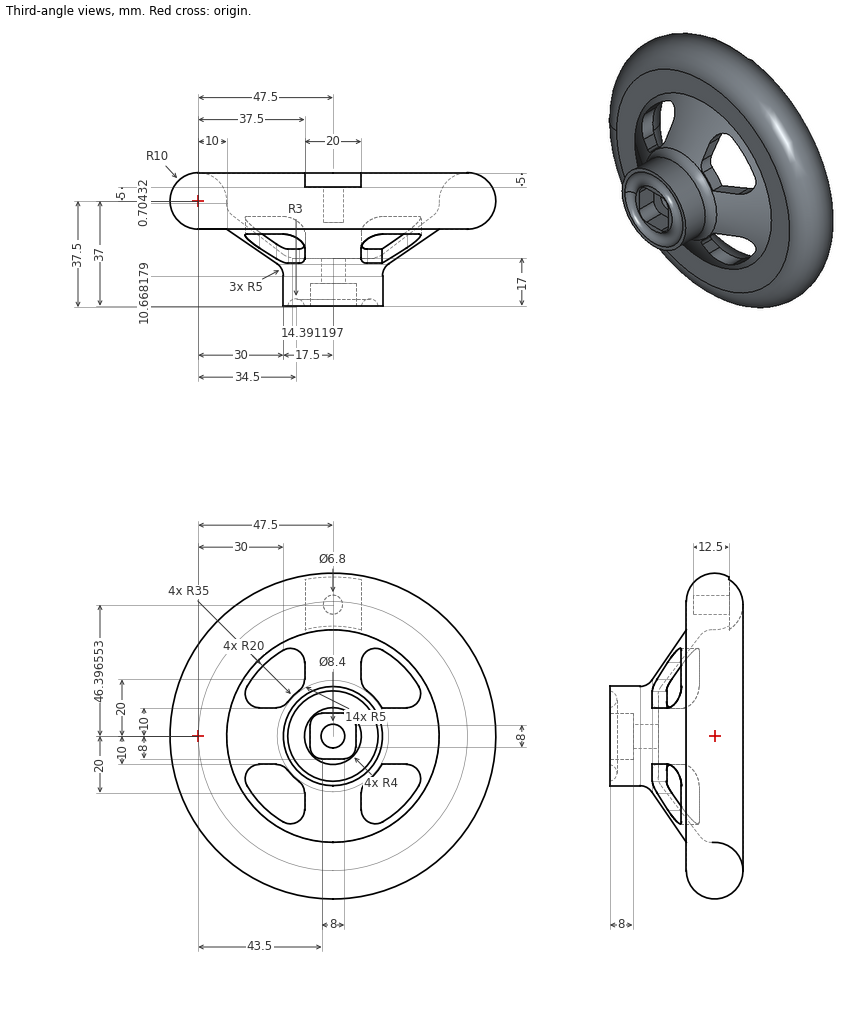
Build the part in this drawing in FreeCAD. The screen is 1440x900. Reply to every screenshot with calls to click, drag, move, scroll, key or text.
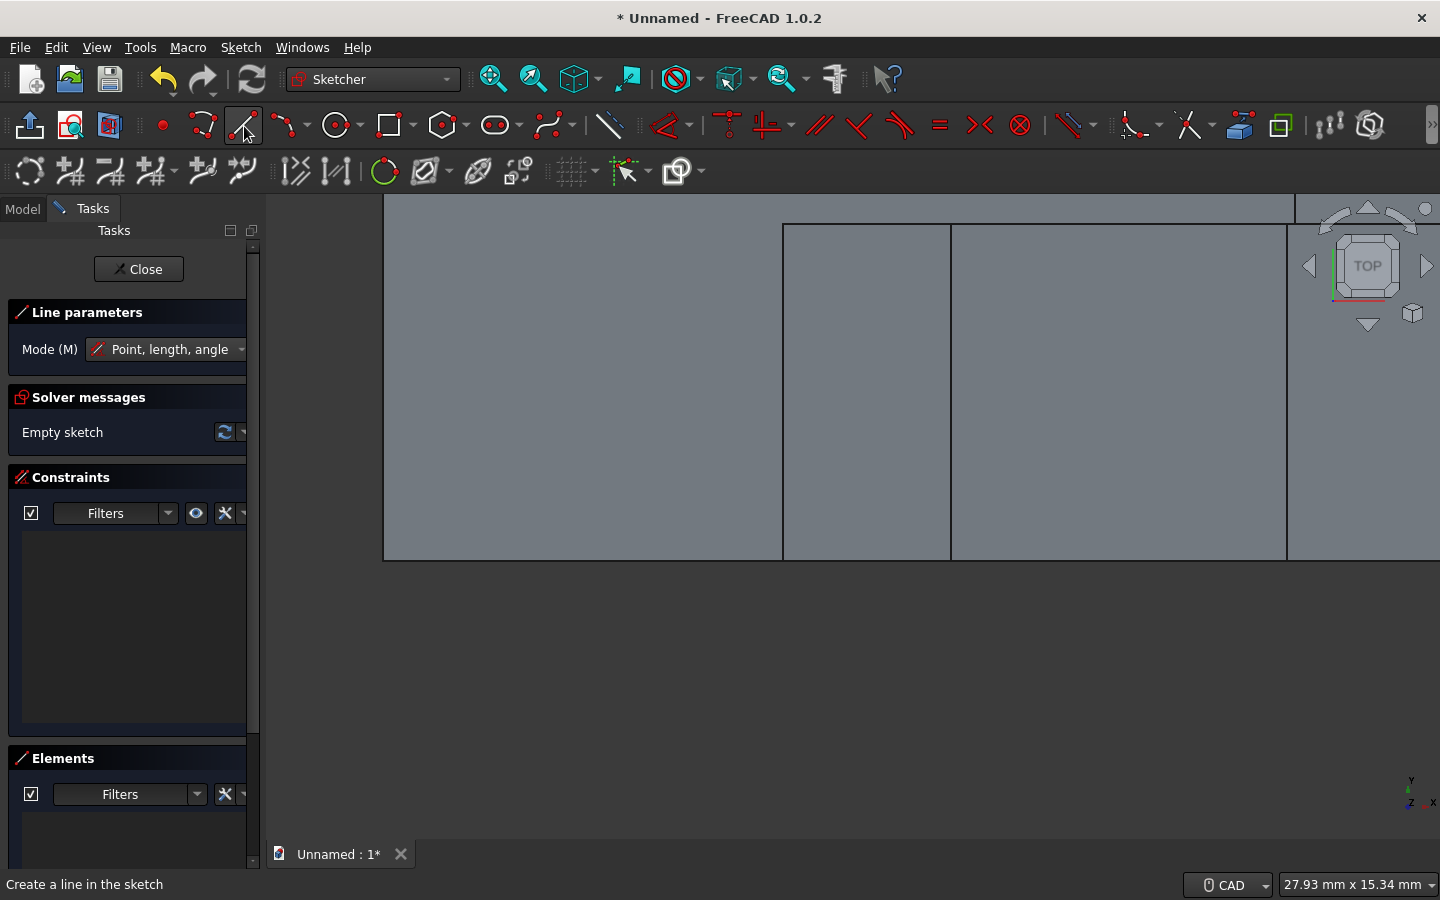
click(448, 561)
click(697, 561)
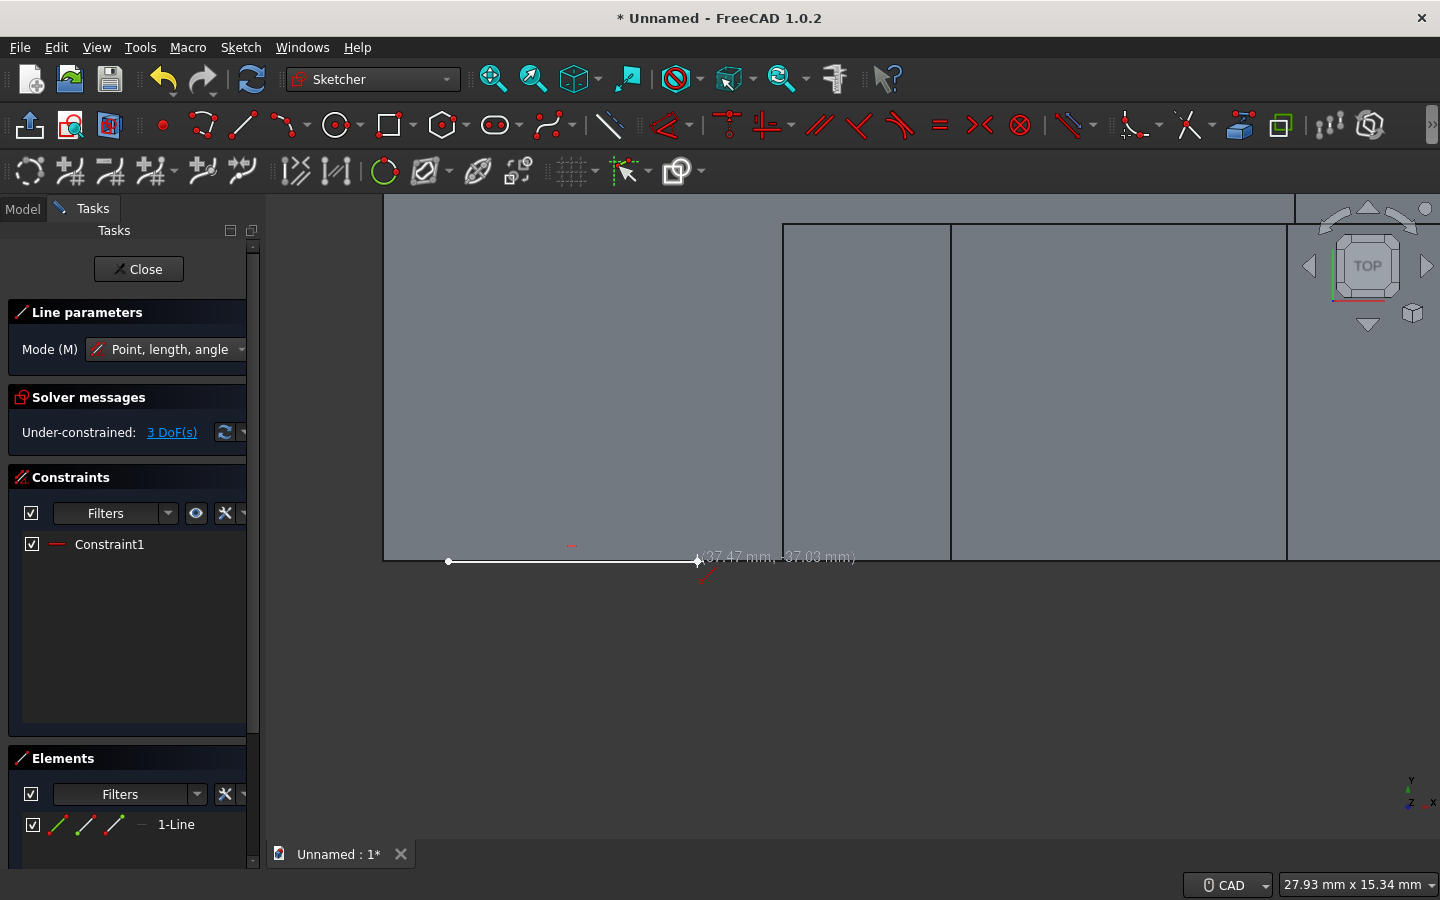
click(284, 126)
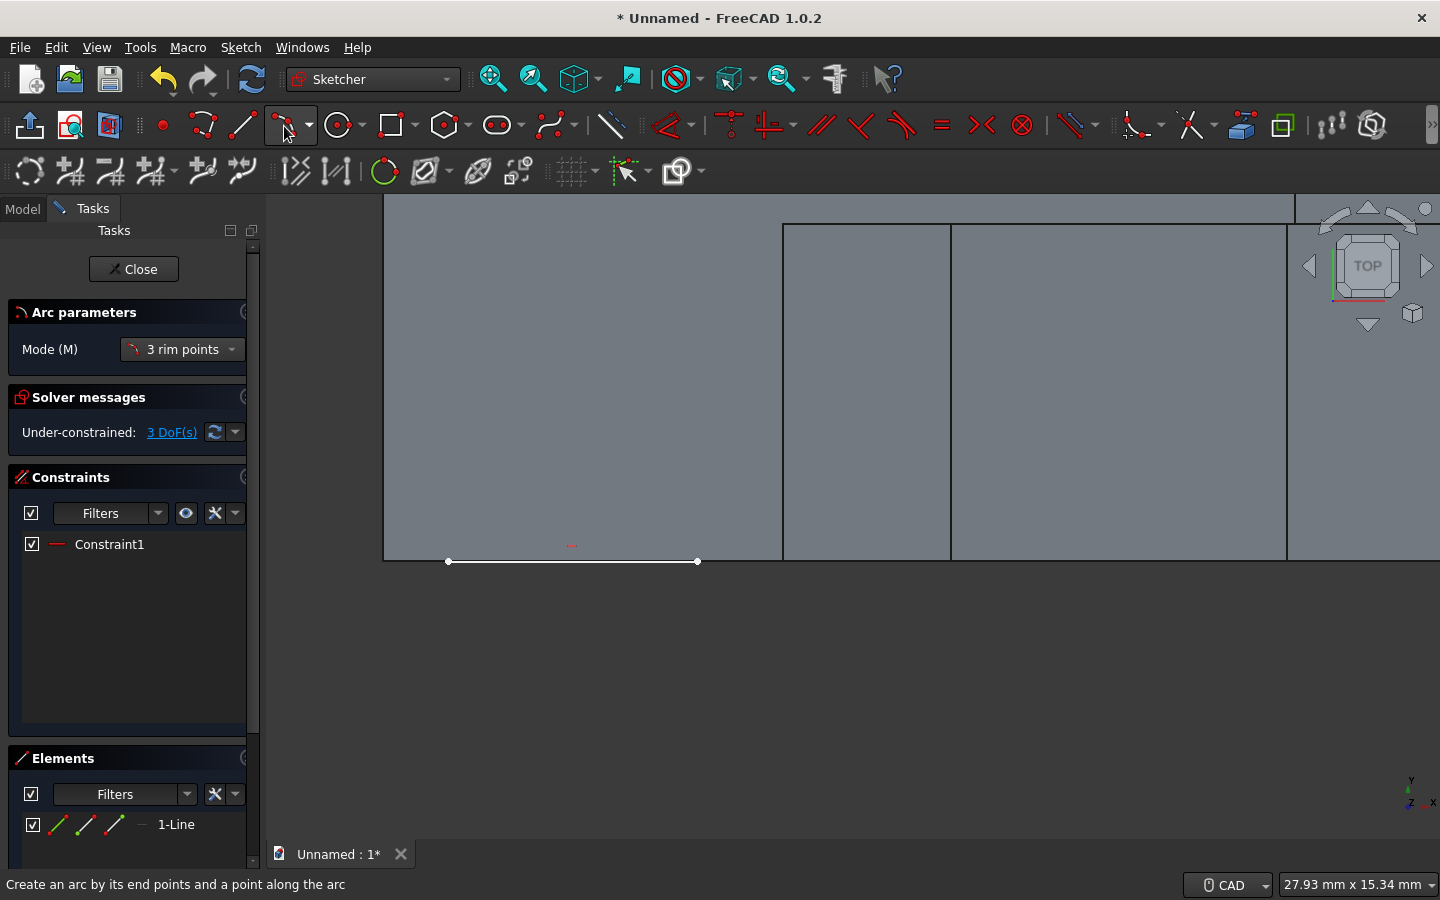
click(697, 562)
click(448, 562)
click(572, 456)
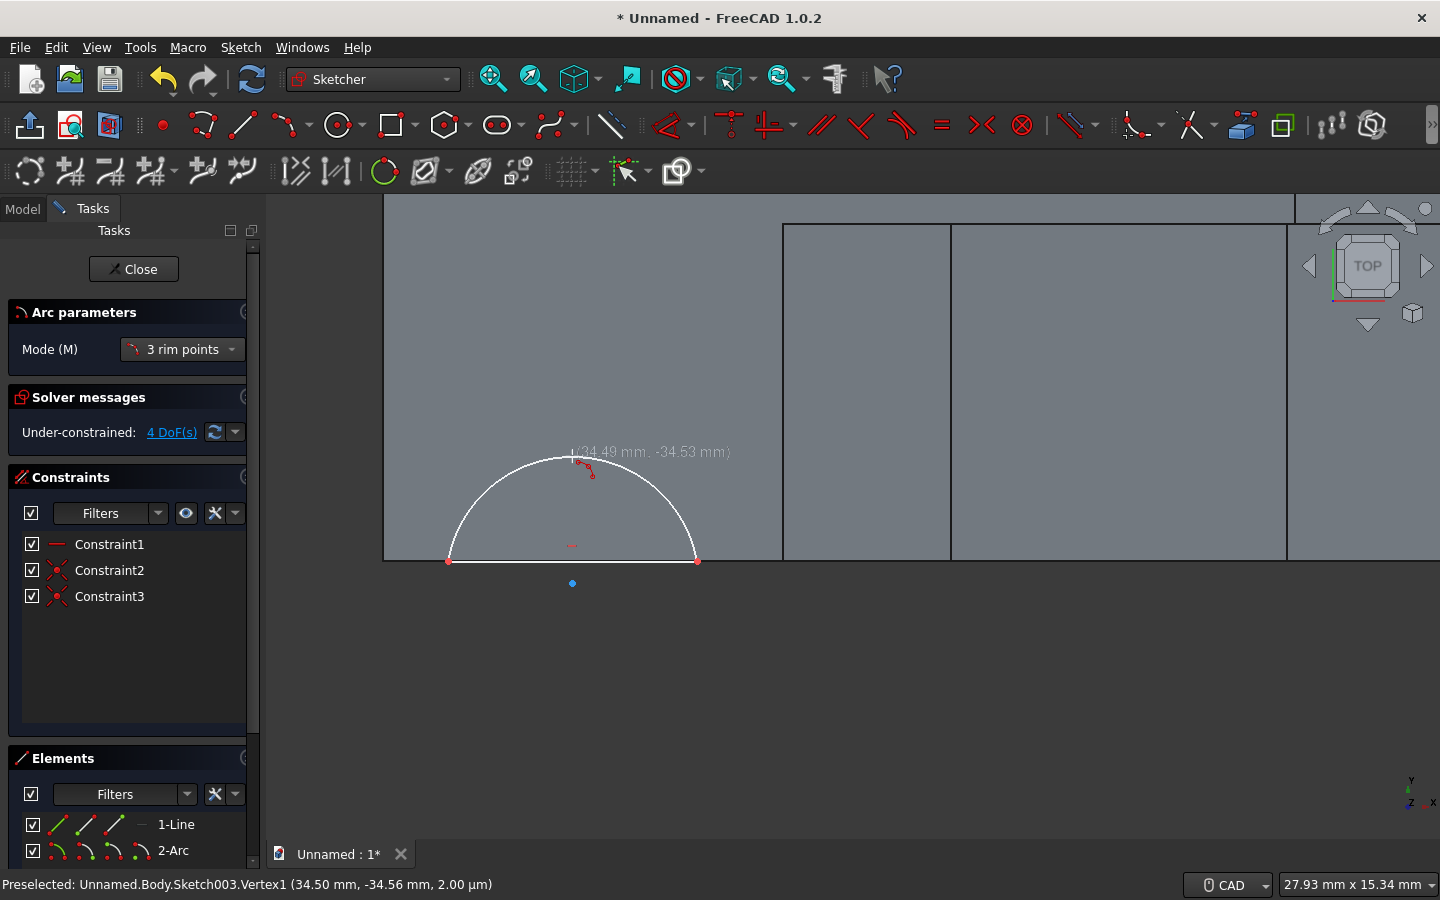
click(244, 126)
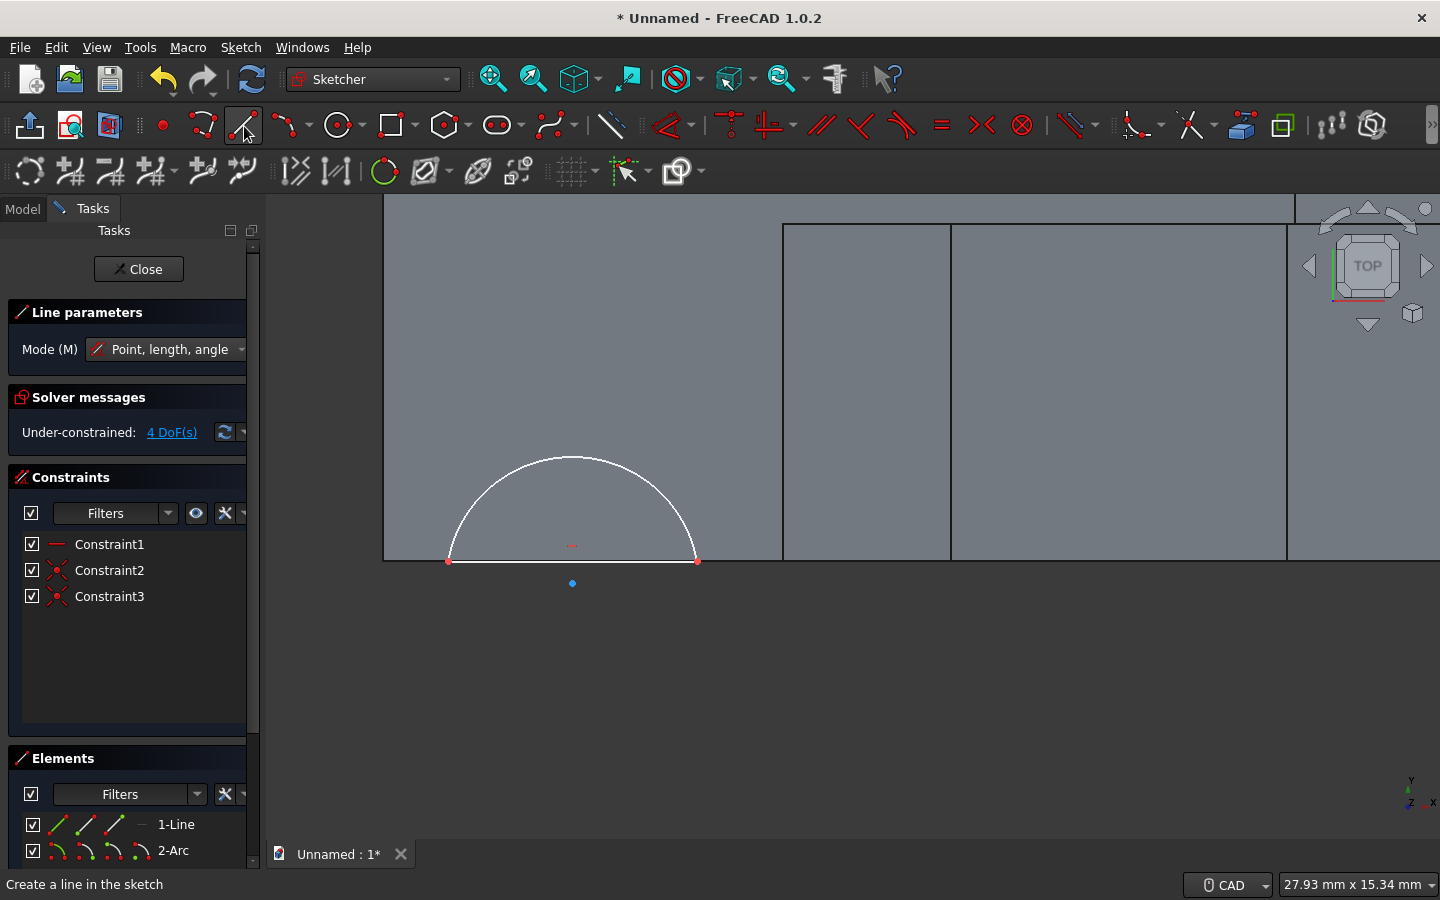
click(1119, 445)
click(1119, 571)
key(Escape)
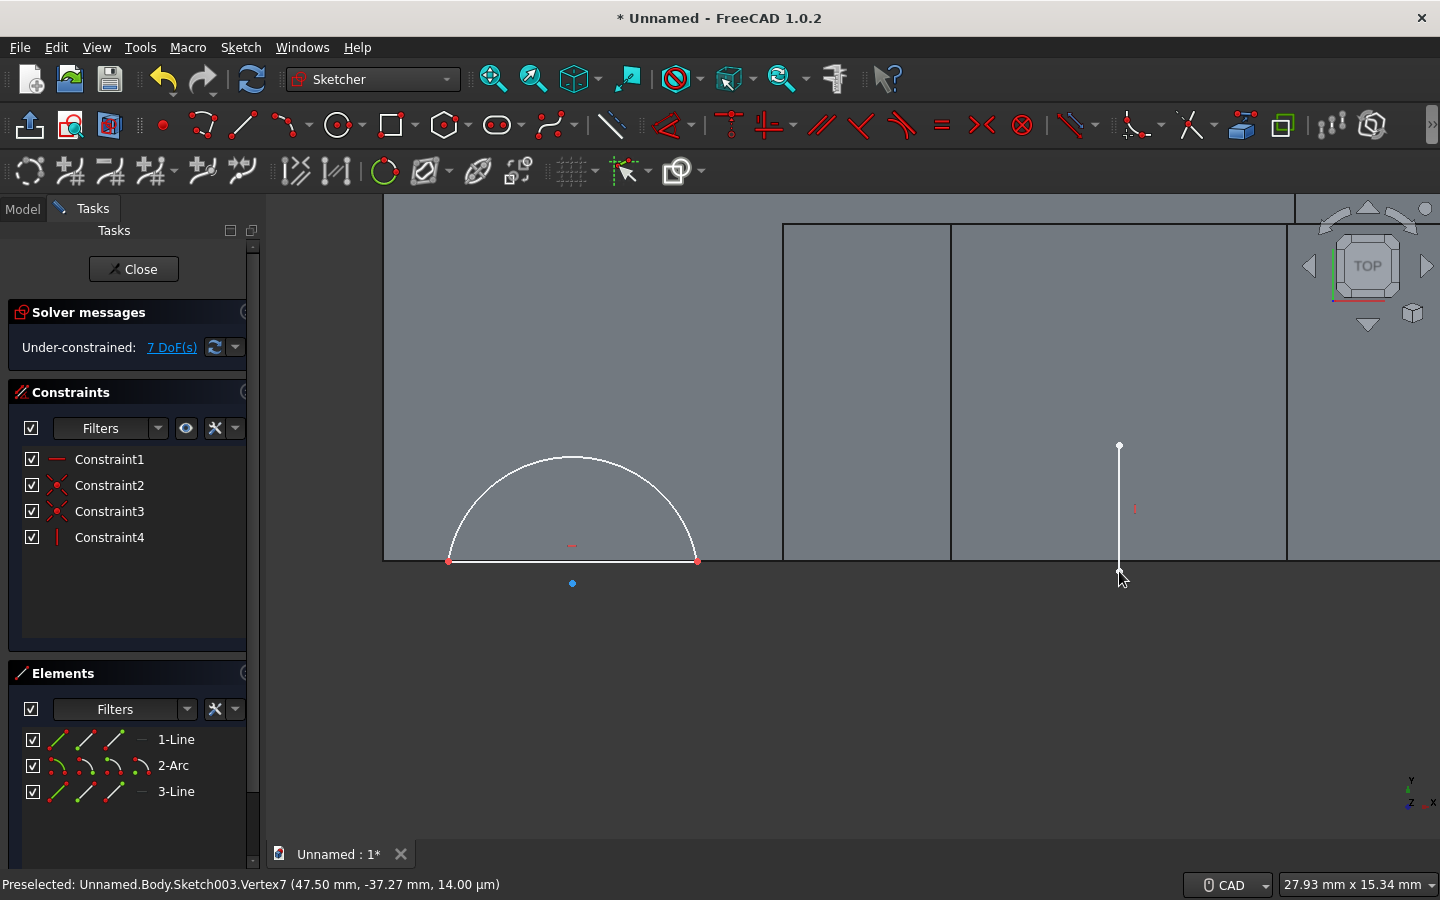
click(1119, 484)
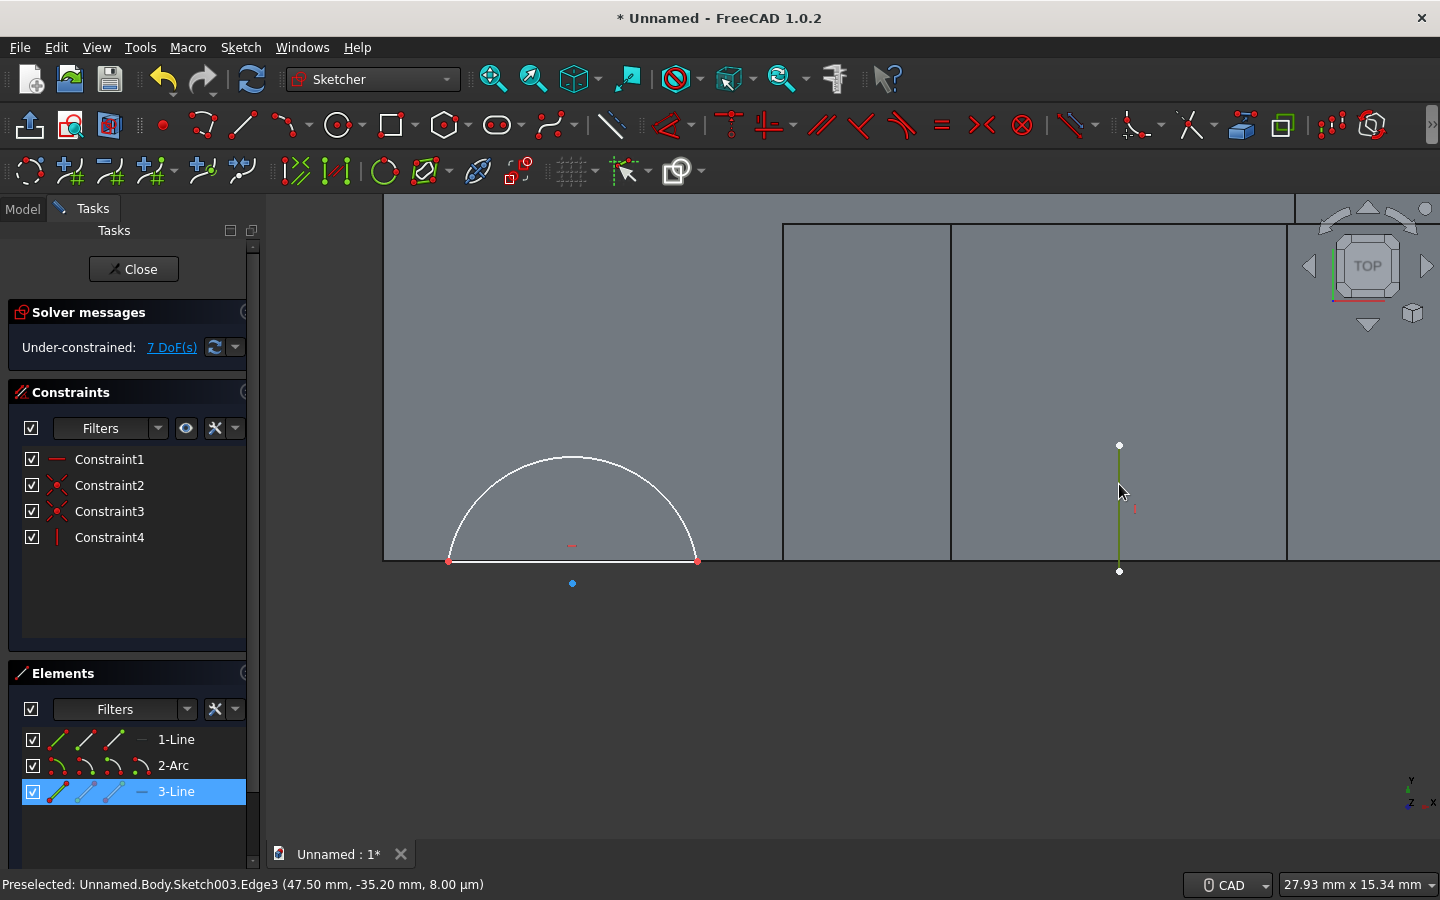
click(612, 126)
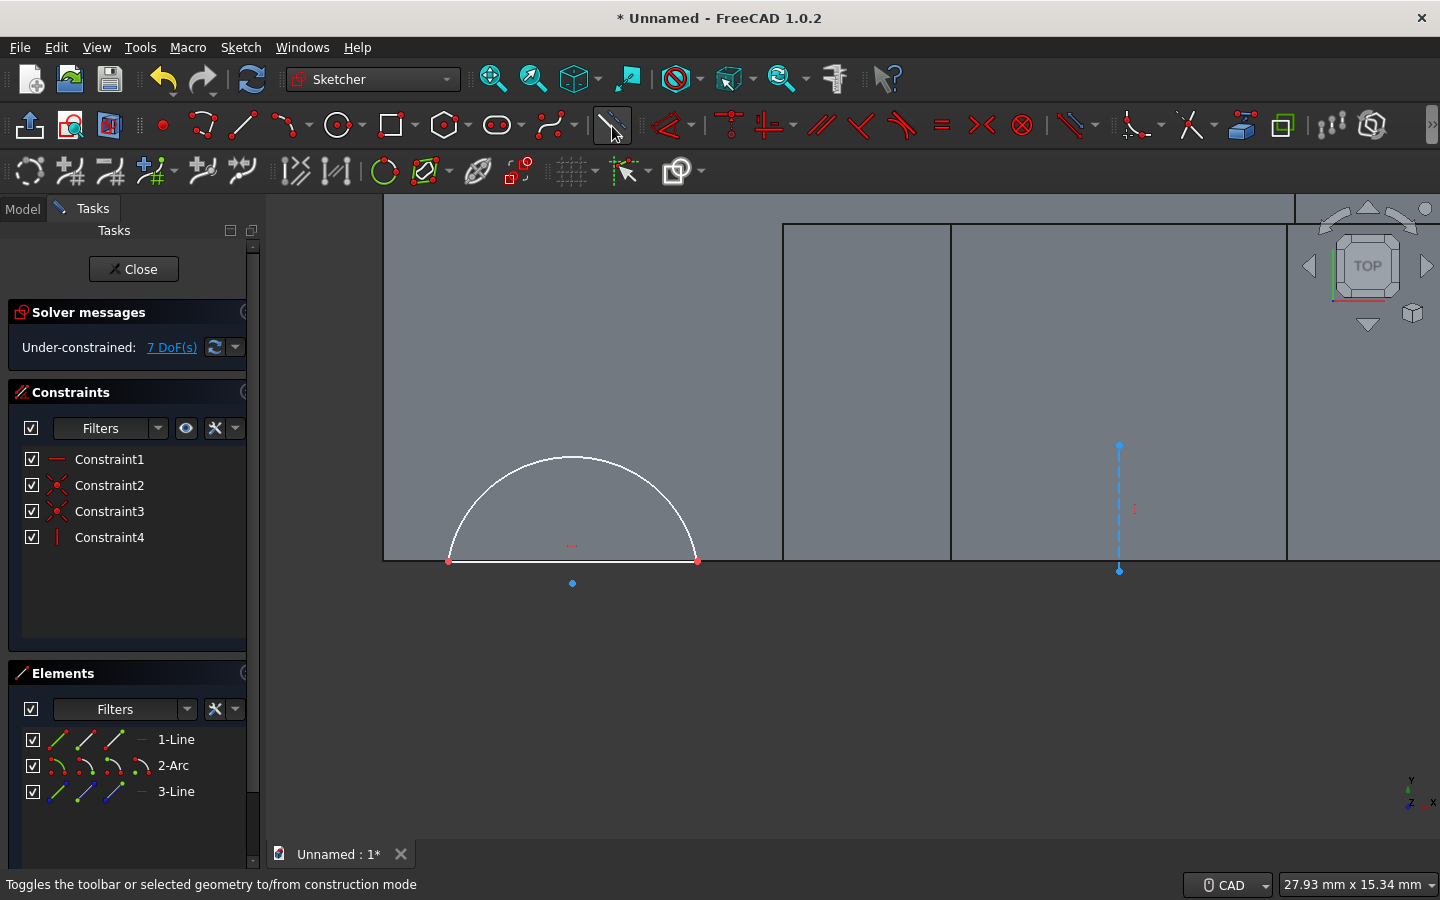
click(666, 126)